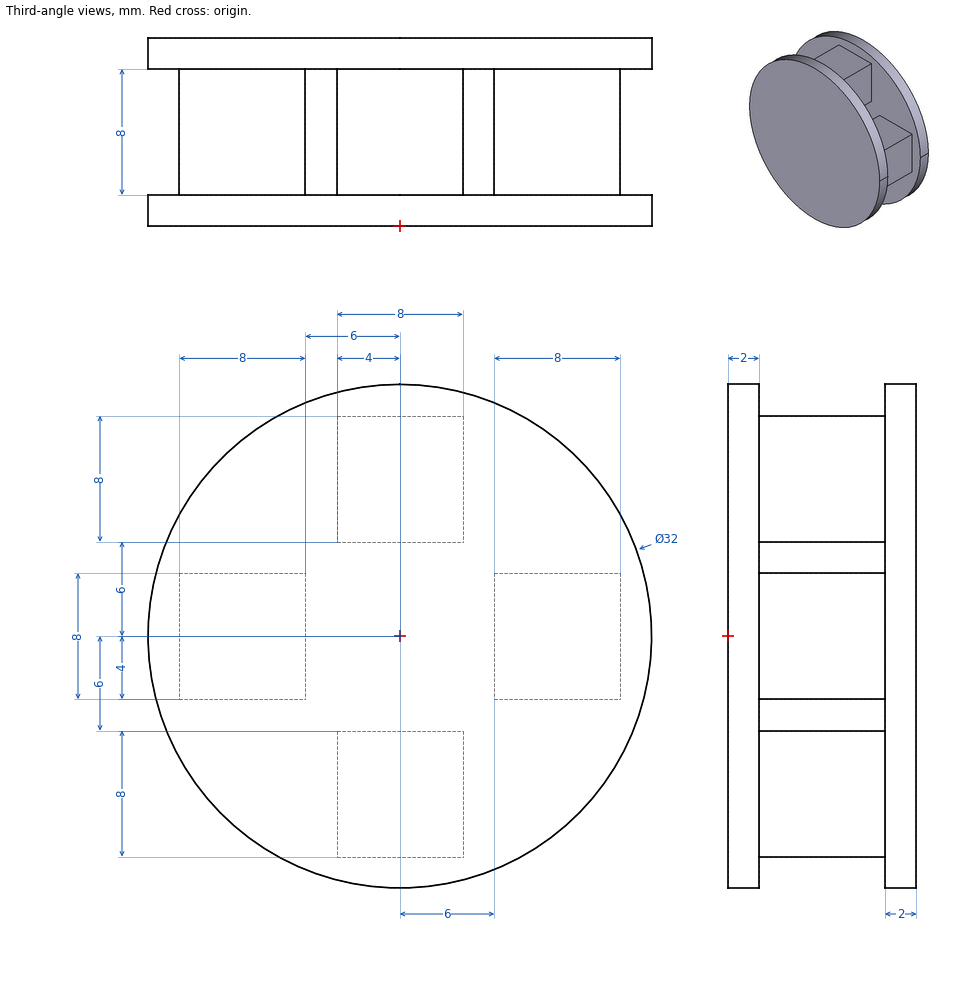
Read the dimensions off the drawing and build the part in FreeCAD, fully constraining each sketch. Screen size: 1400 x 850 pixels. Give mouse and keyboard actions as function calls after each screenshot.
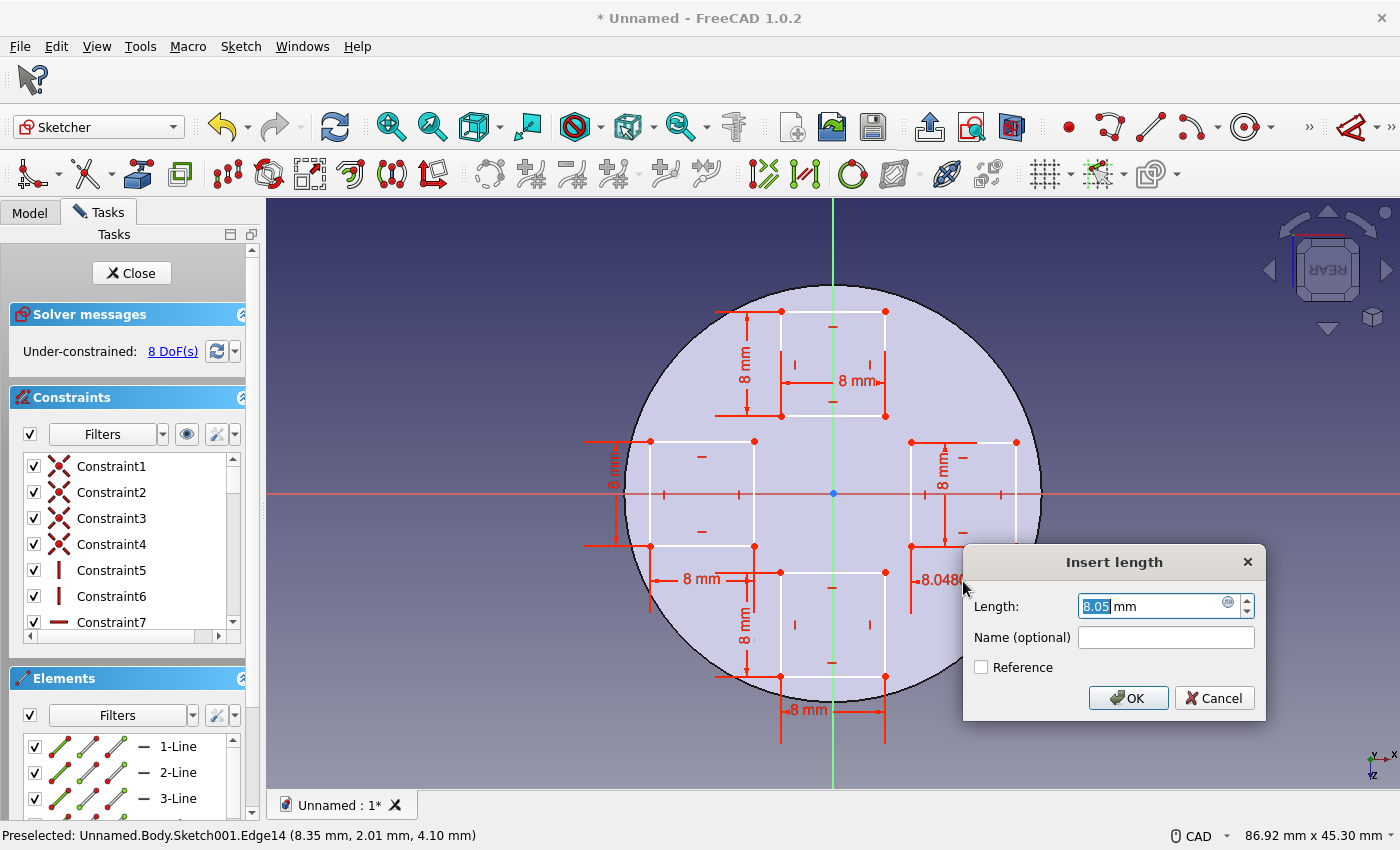
text(8)
key(Return)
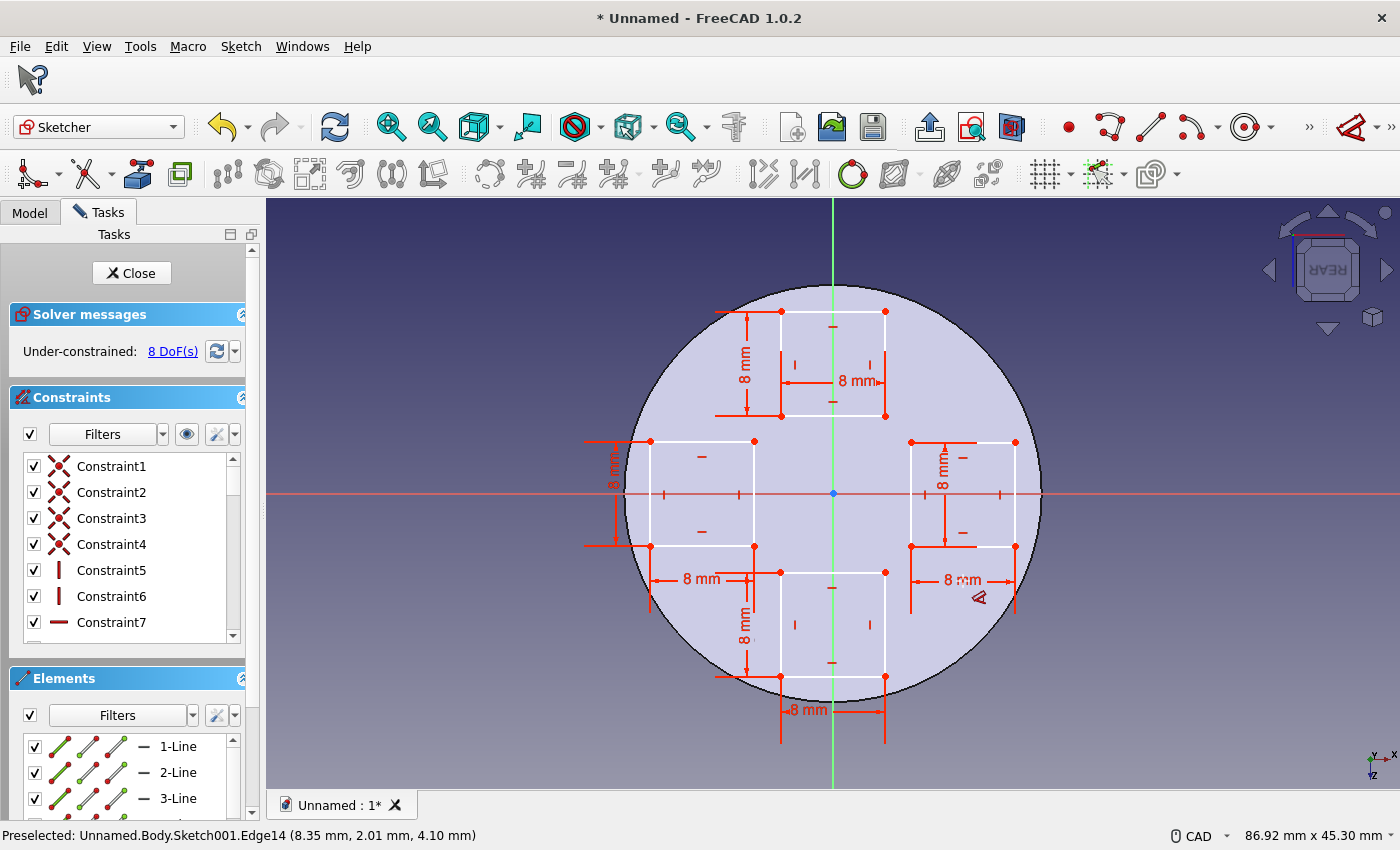
click(650, 442)
click(616, 450)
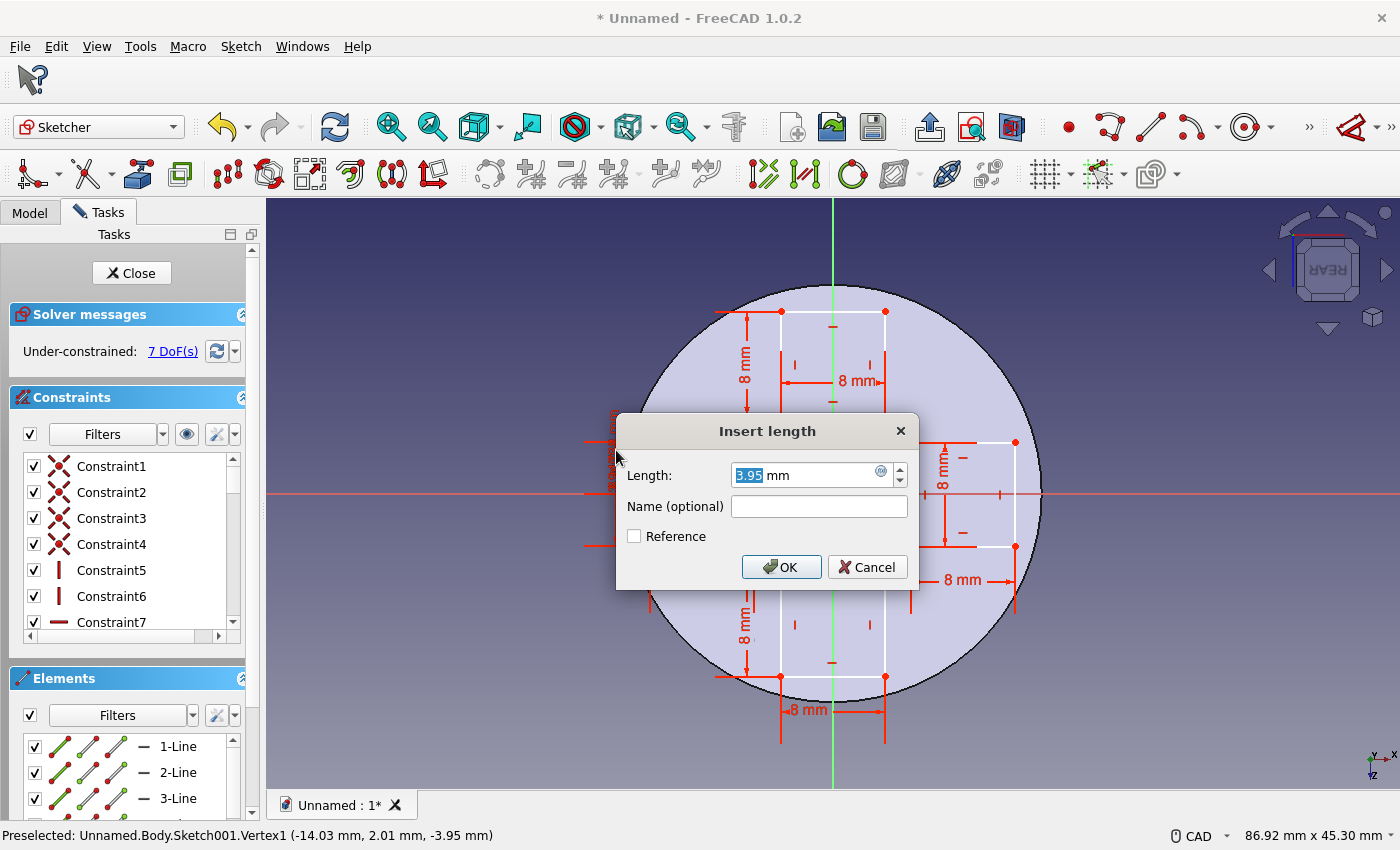
text(4)
key(Return)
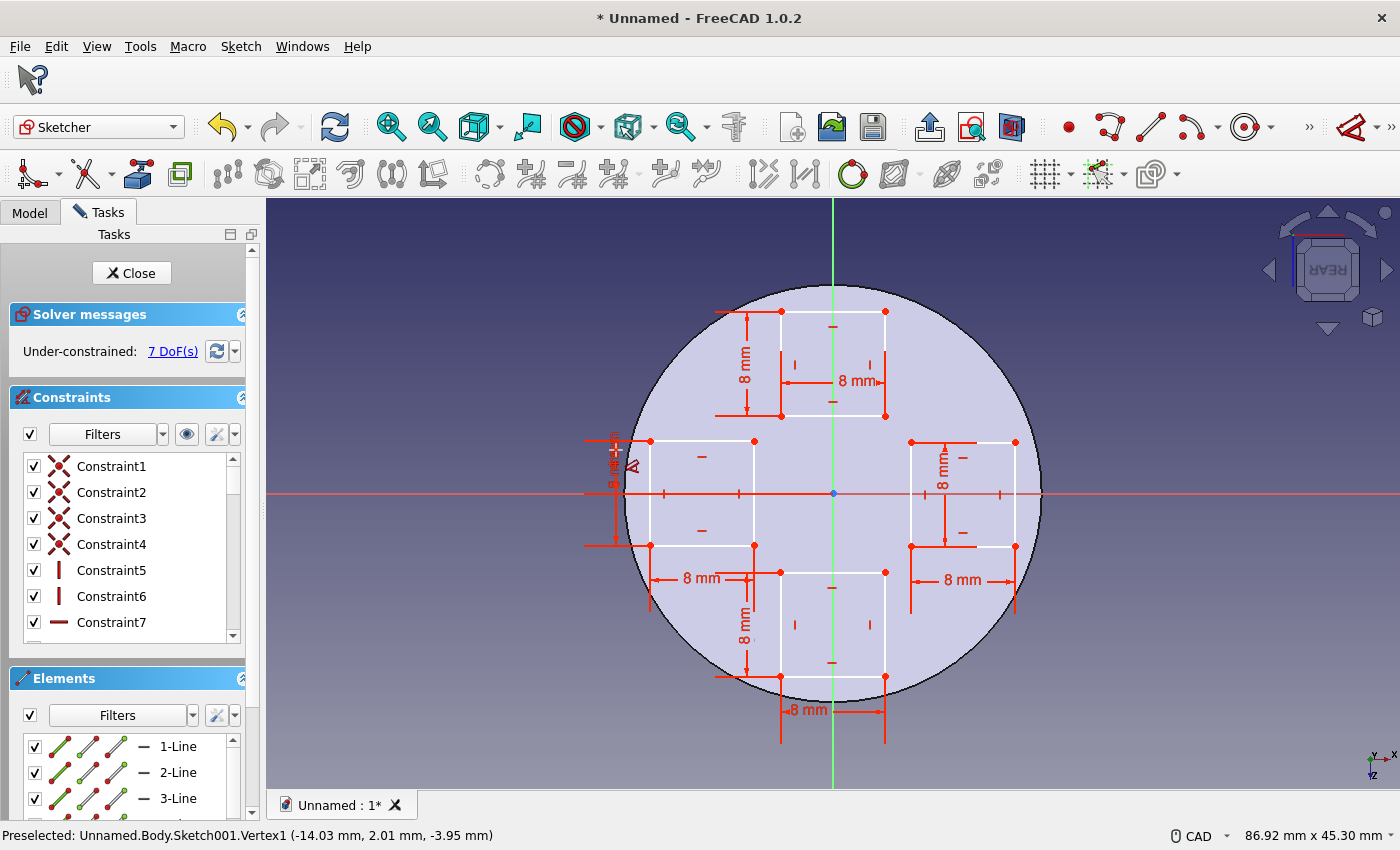
click(754, 546)
click(794, 460)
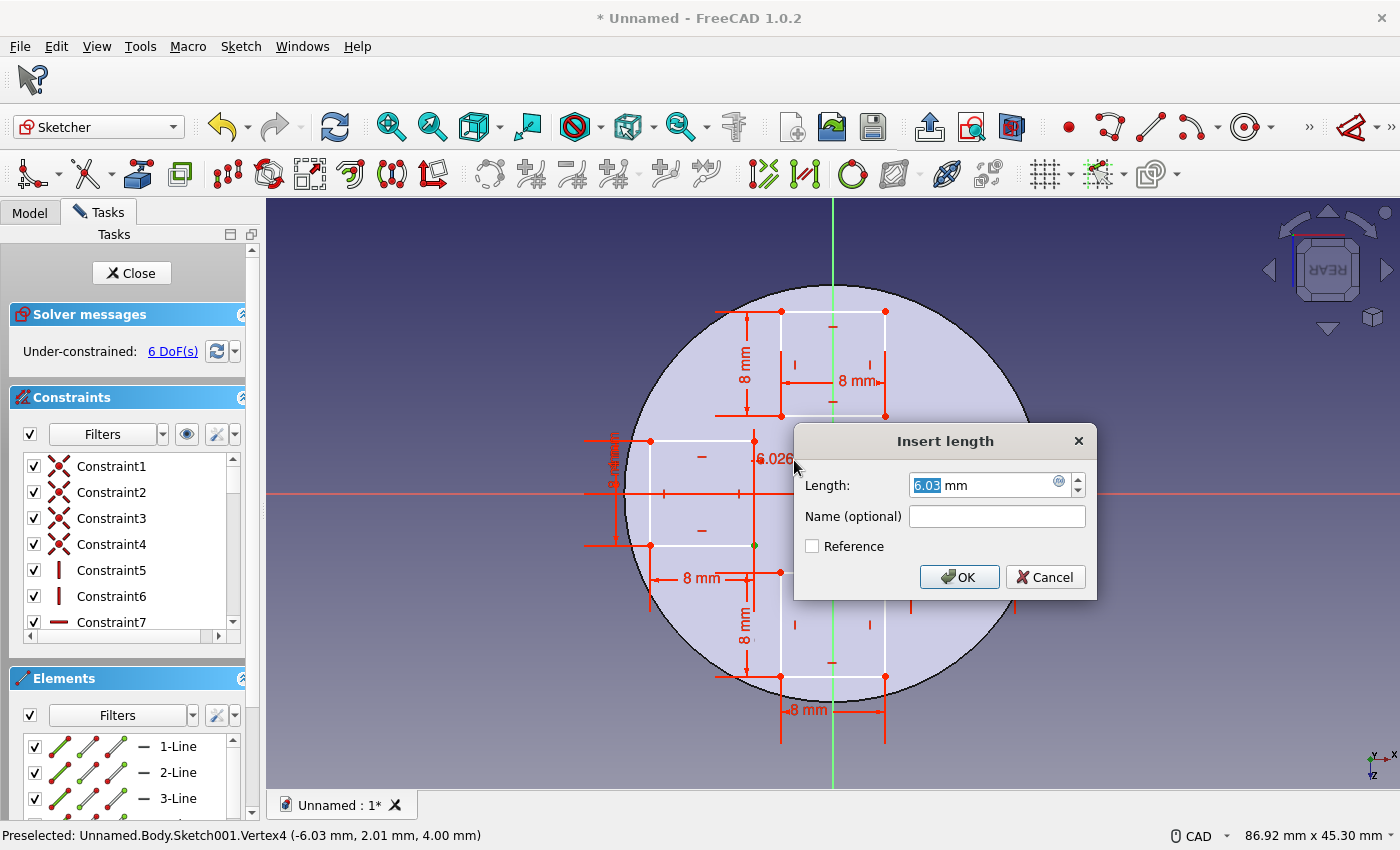
text(6)
key(Return)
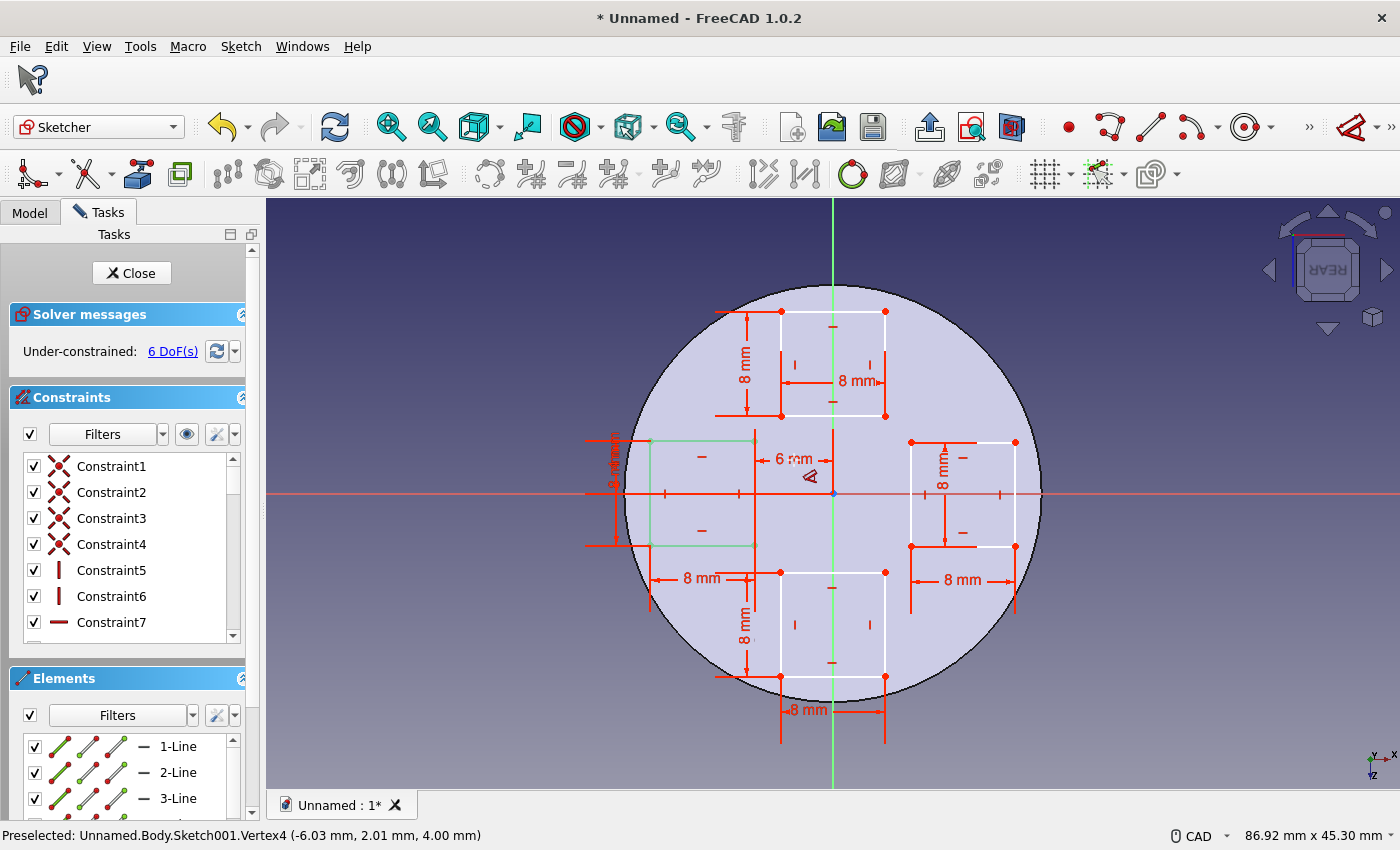
click(781, 573)
click(819, 607)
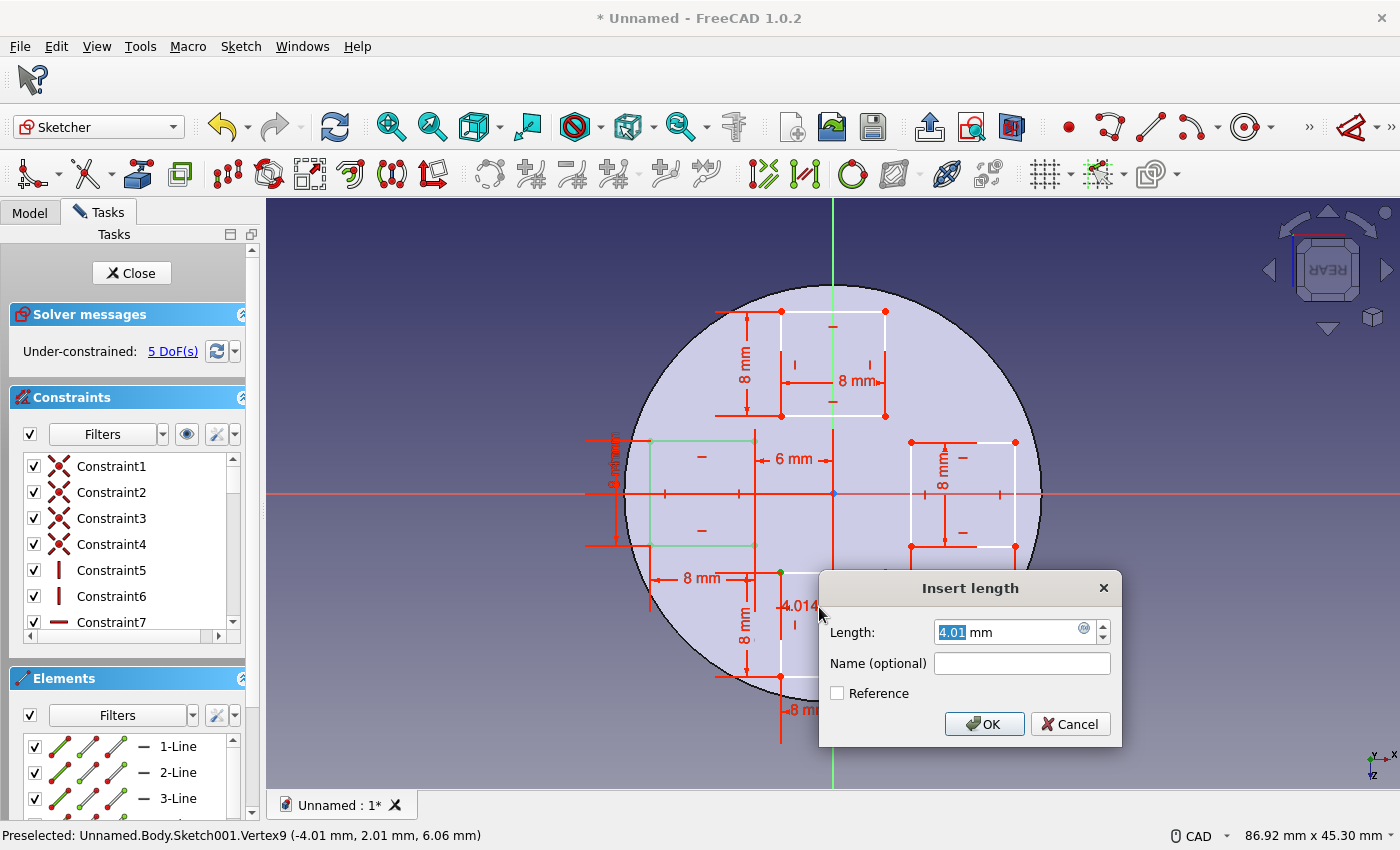
text(4)
key(Return)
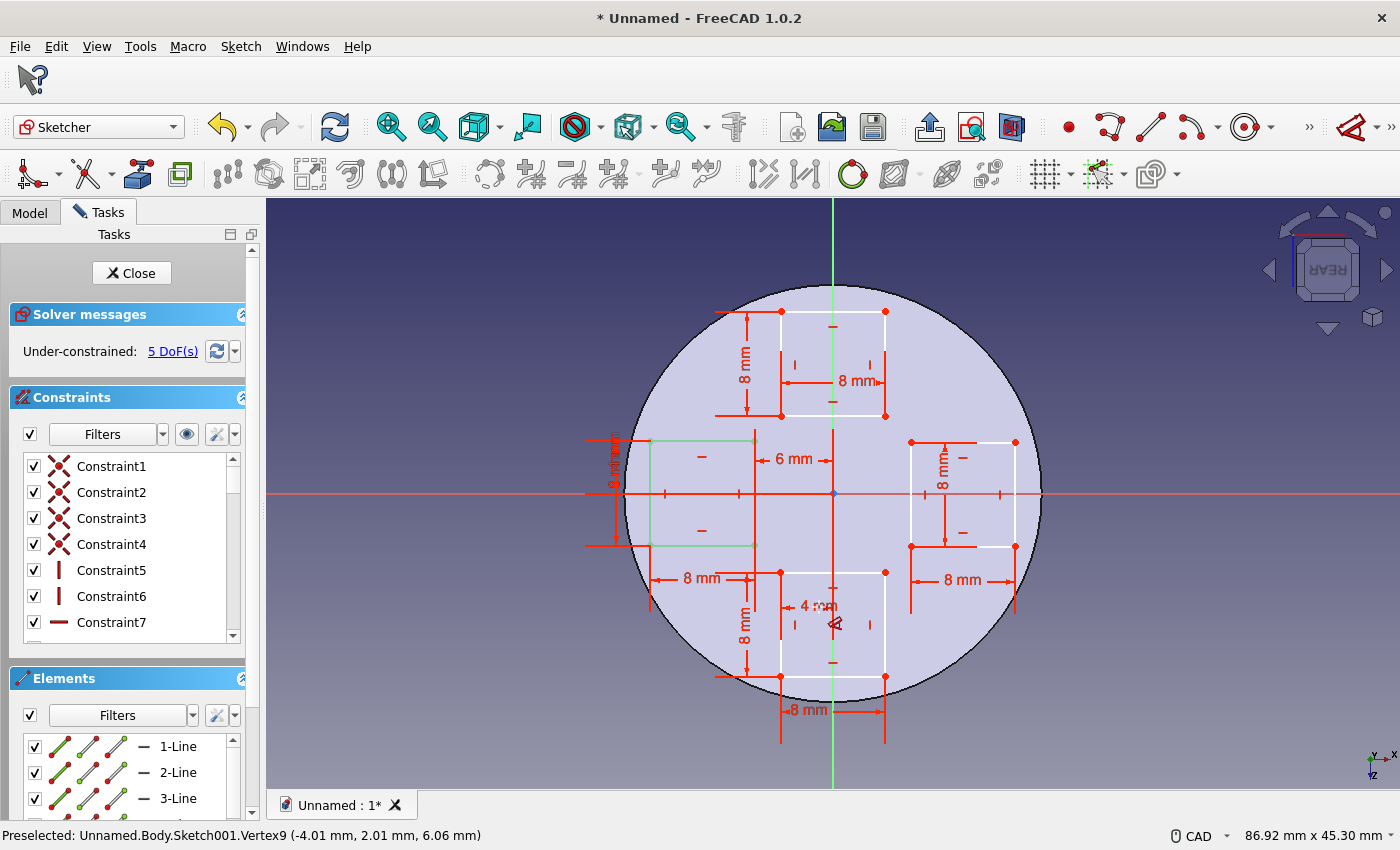
click(781, 573)
click(867, 533)